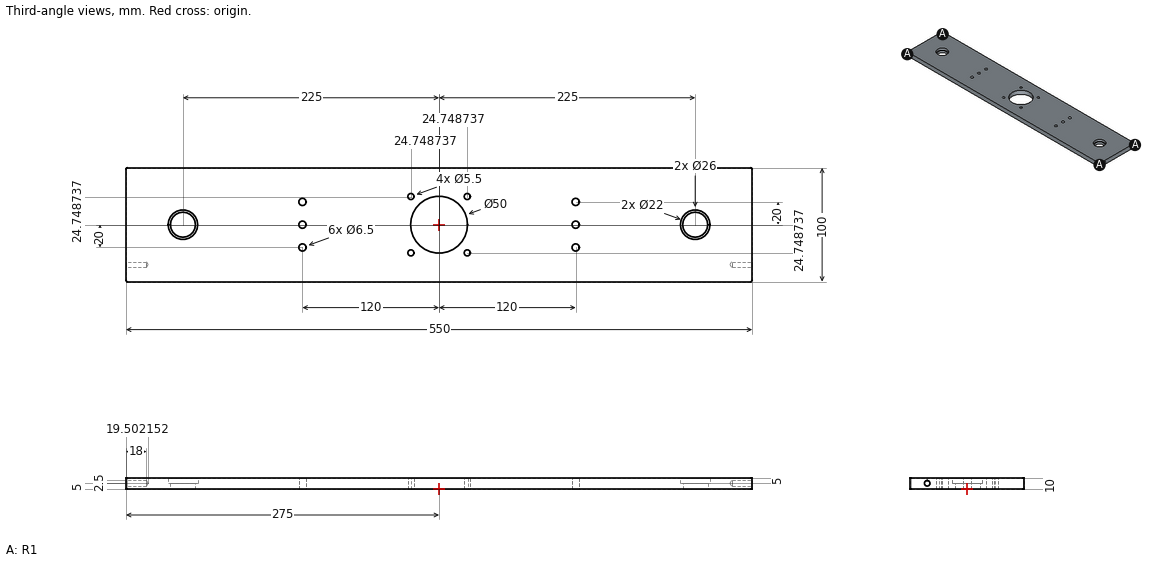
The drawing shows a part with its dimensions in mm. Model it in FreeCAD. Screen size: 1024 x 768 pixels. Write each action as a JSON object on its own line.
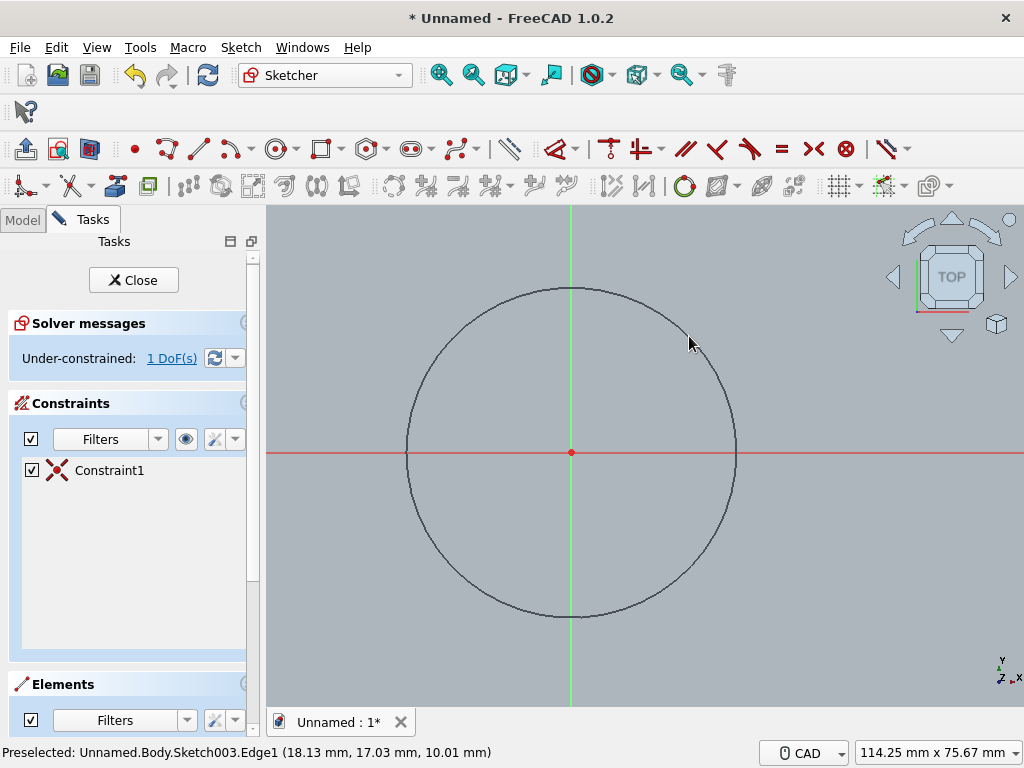
{"action": "key", "text": "d"}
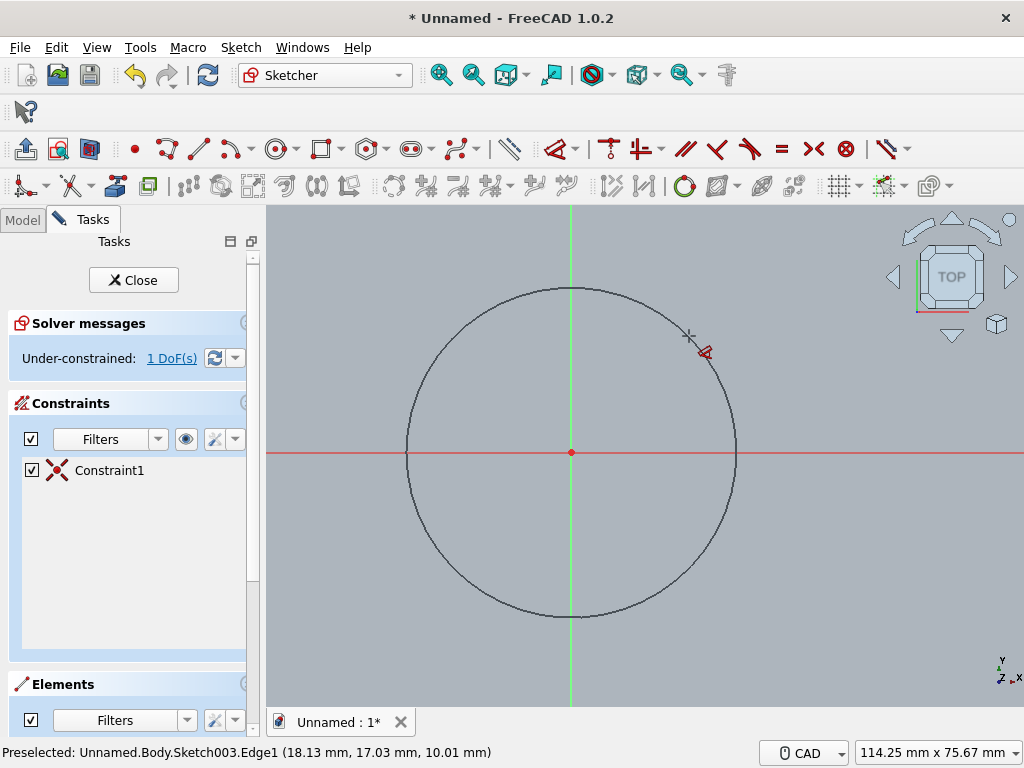
{"action": "left_click", "coordinate": [688, 336]}
{"action": "left_click", "coordinate": [711, 313]}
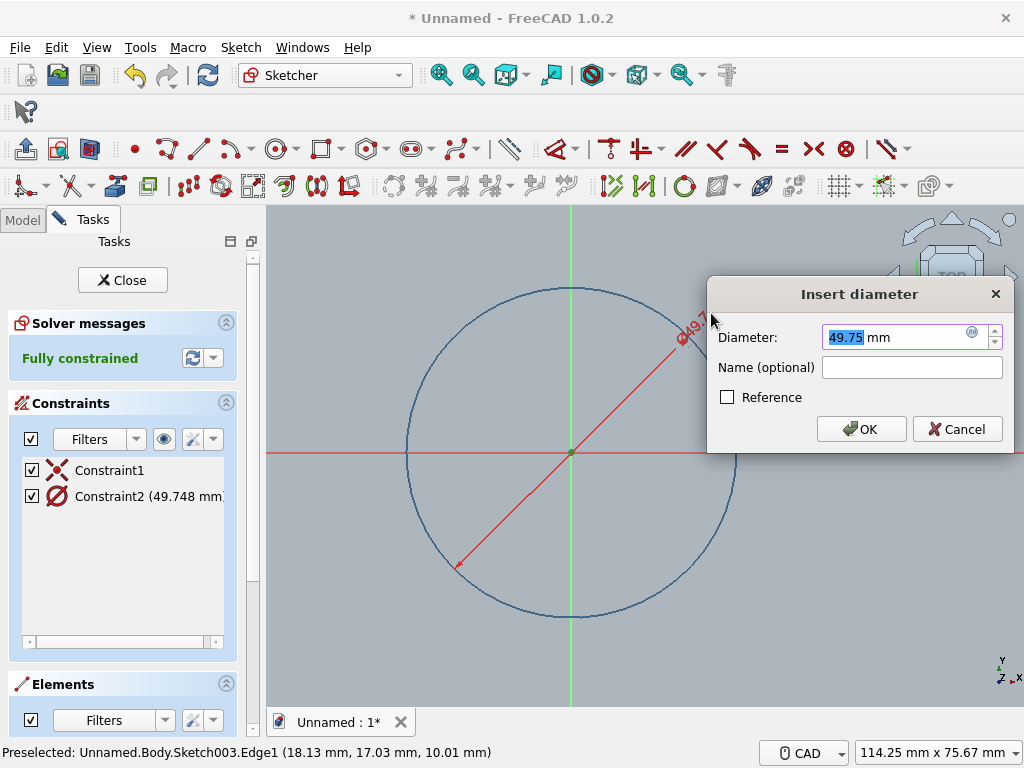
{"action": "type", "text": "50"}
{"action": "key", "text": "Return"}
{"action": "key", "text": "Escape"}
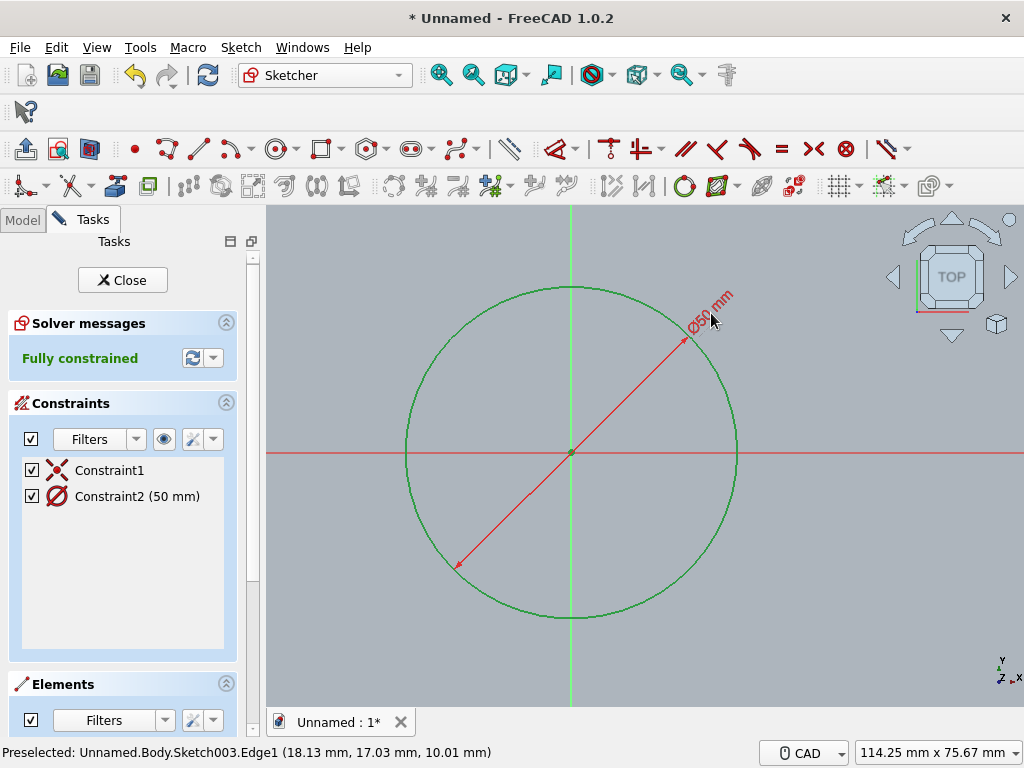
{"action": "left_click", "coordinate": [123, 280]}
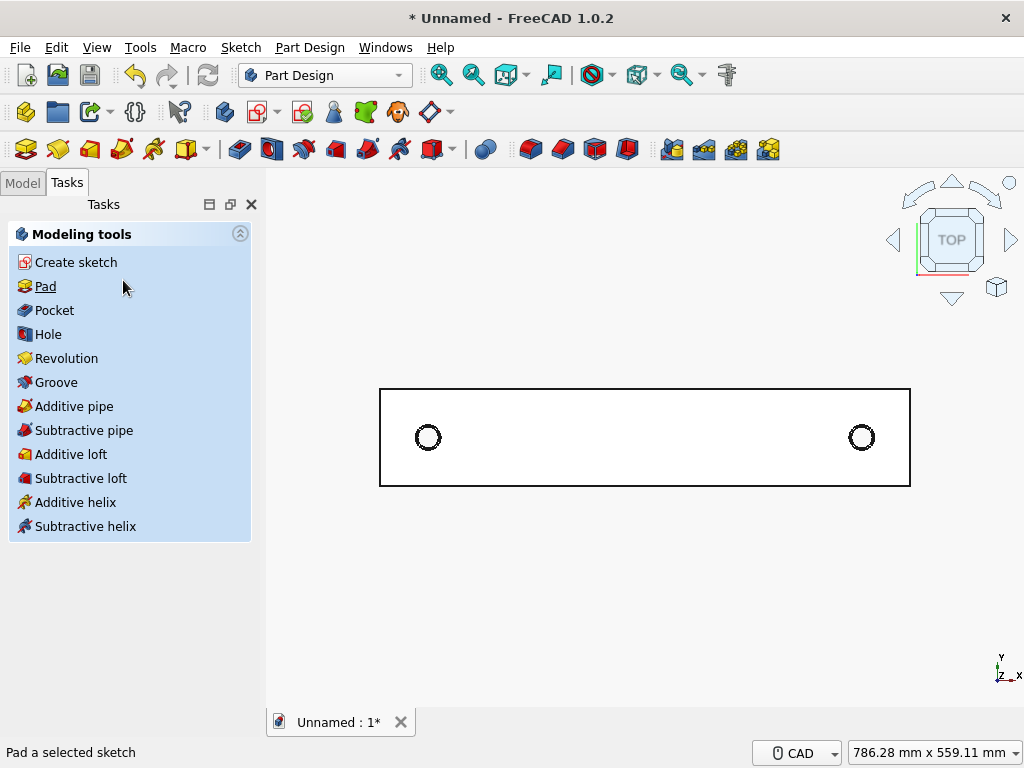
{"action": "left_click", "coordinate": [240, 150]}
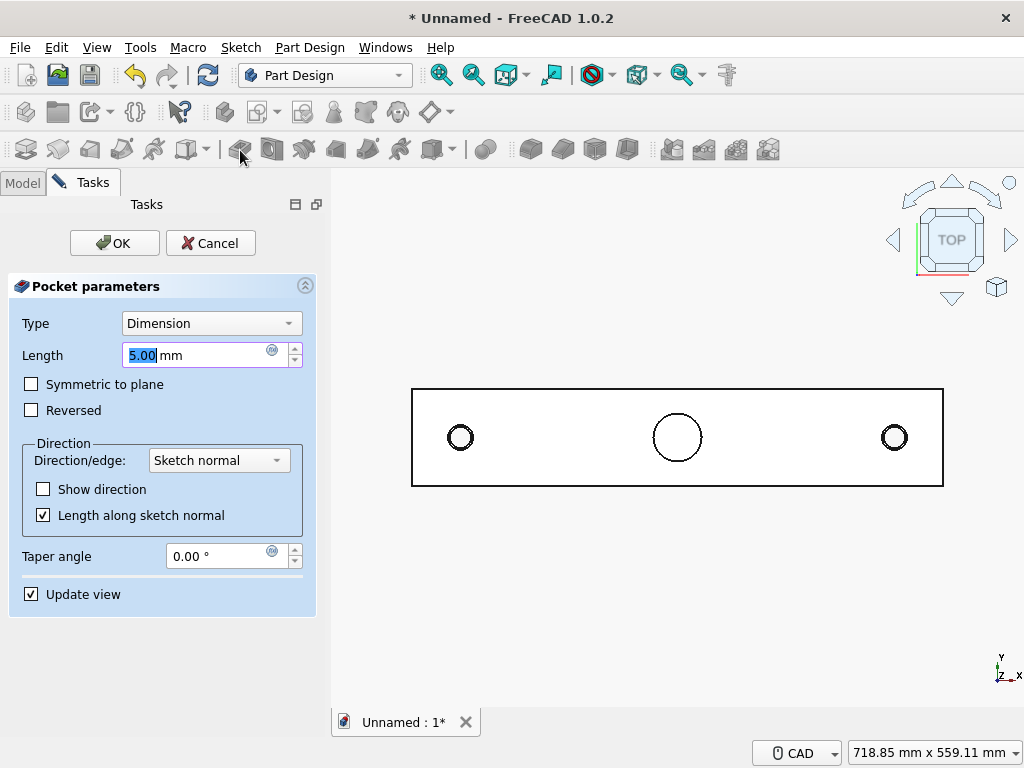
{"action": "left_click", "coordinate": [212, 324]}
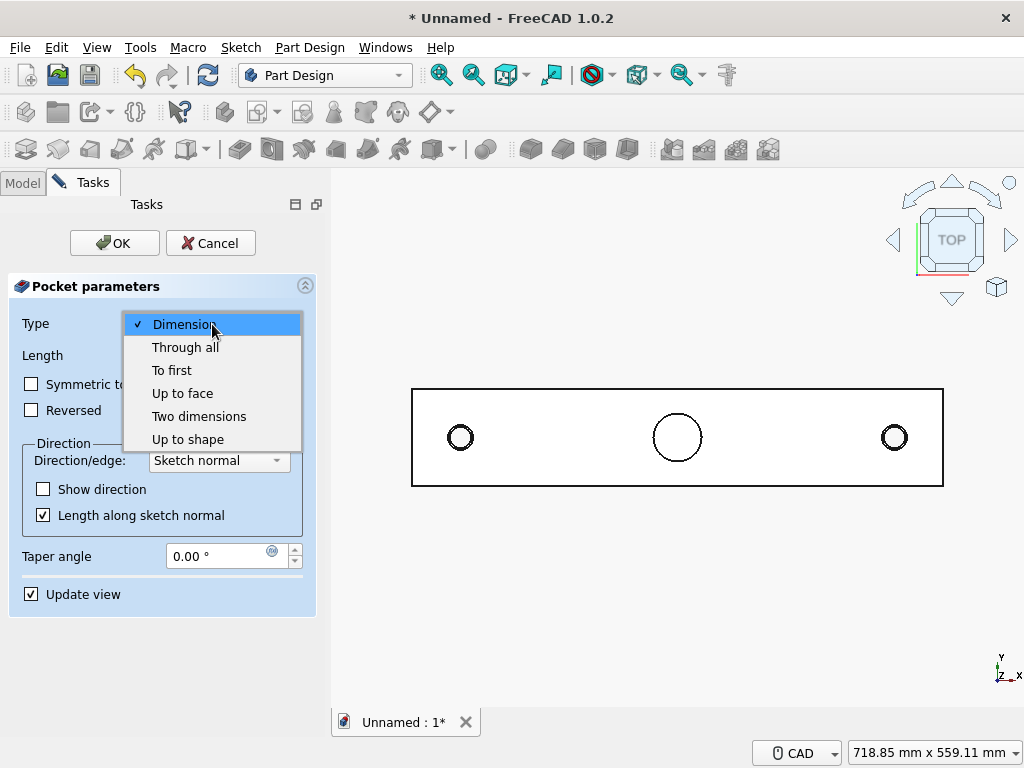
{"action": "left_click", "coordinate": [212, 348]}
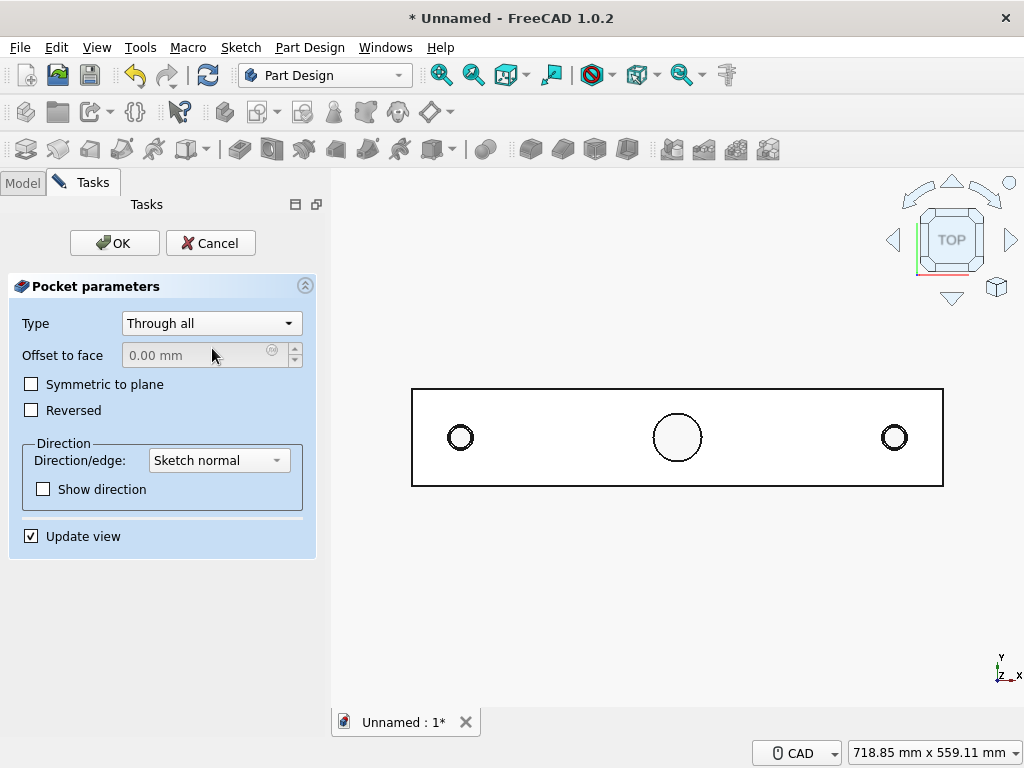
{"action": "left_click", "coordinate": [115, 243]}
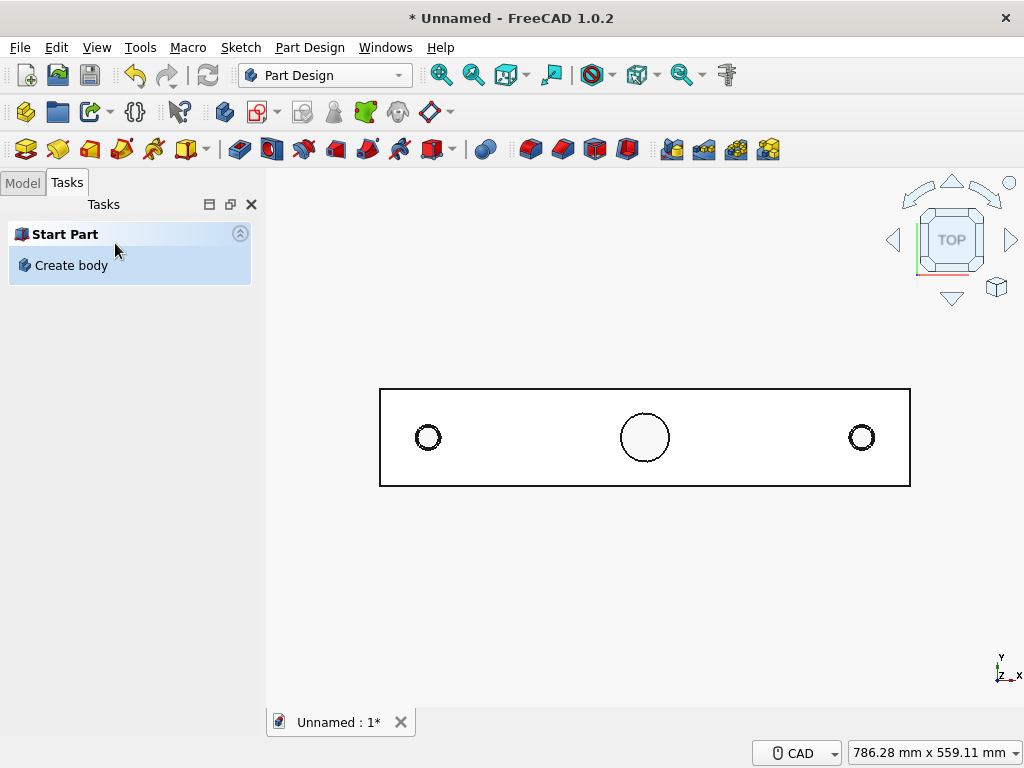
{"action": "left_click", "coordinate": [796, 437]}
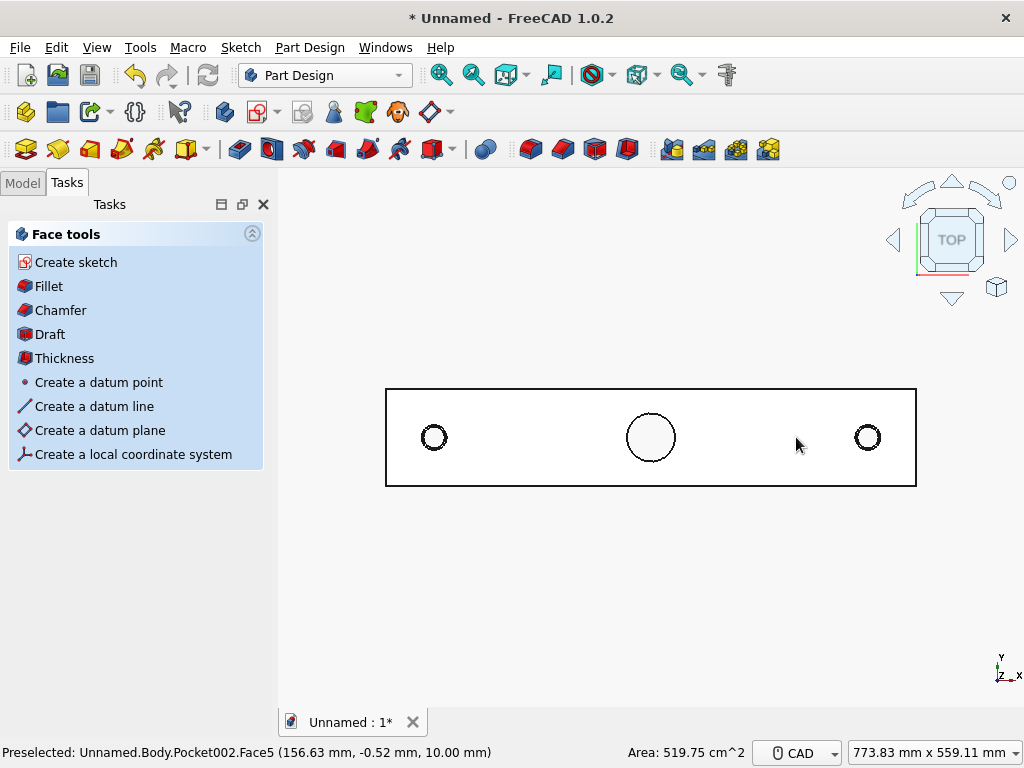
{"action": "left_click", "coordinate": [258, 112]}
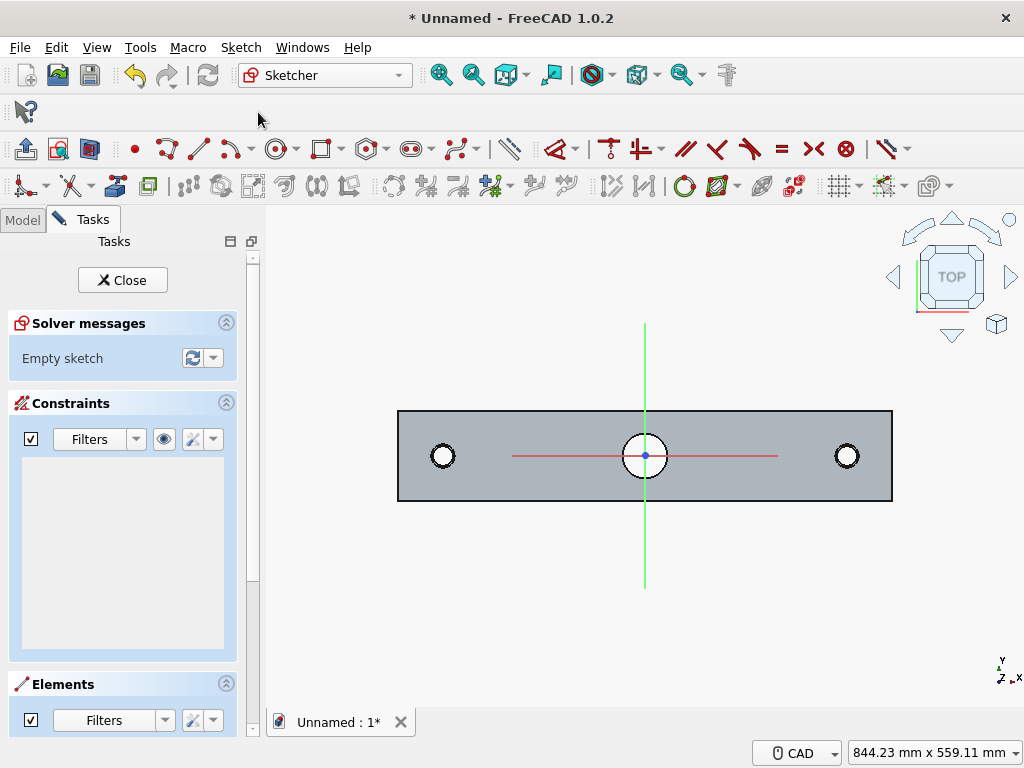
{"action": "scroll", "coordinate": [659, 456], "scroll_direction": "up", "scroll_amount": 9}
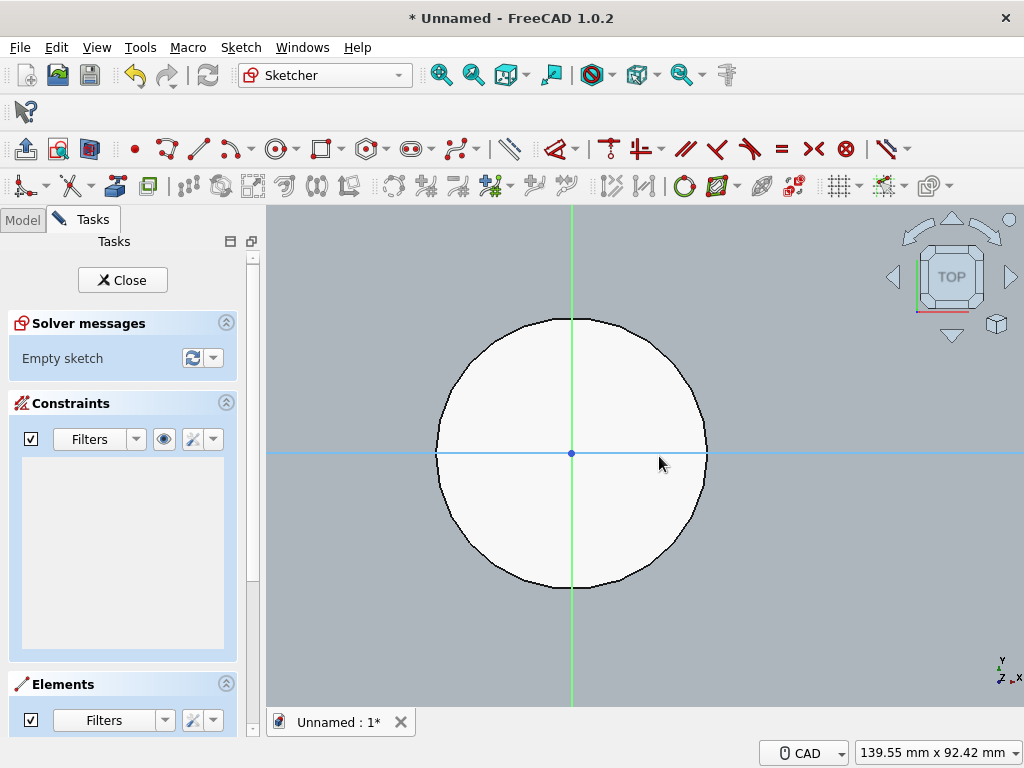
{"action": "key", "text": "g c"}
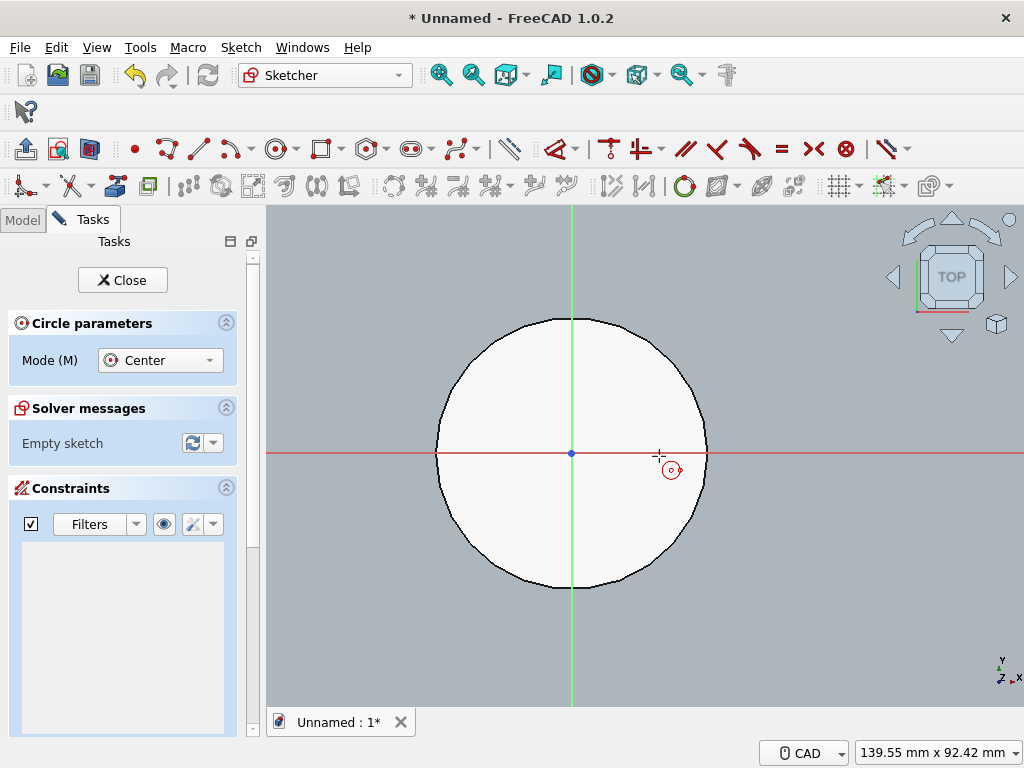
{"action": "scroll", "coordinate": [437, 319], "scroll_direction": "up", "scroll_amount": 3}